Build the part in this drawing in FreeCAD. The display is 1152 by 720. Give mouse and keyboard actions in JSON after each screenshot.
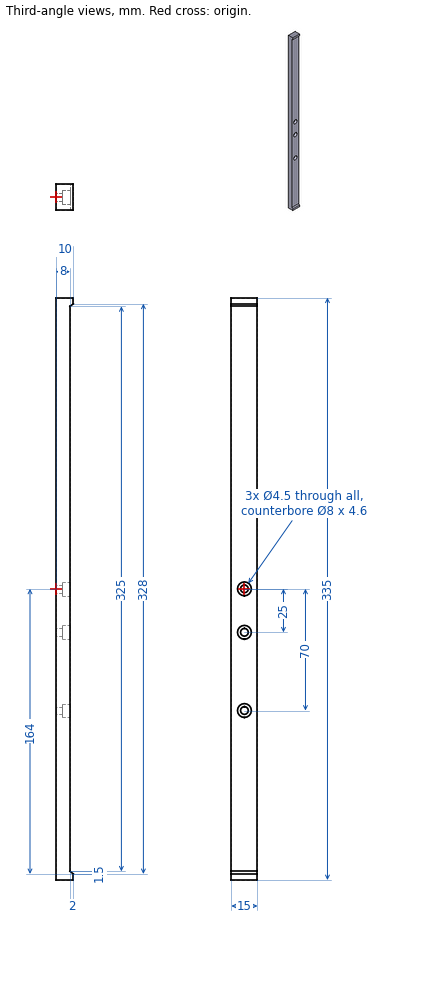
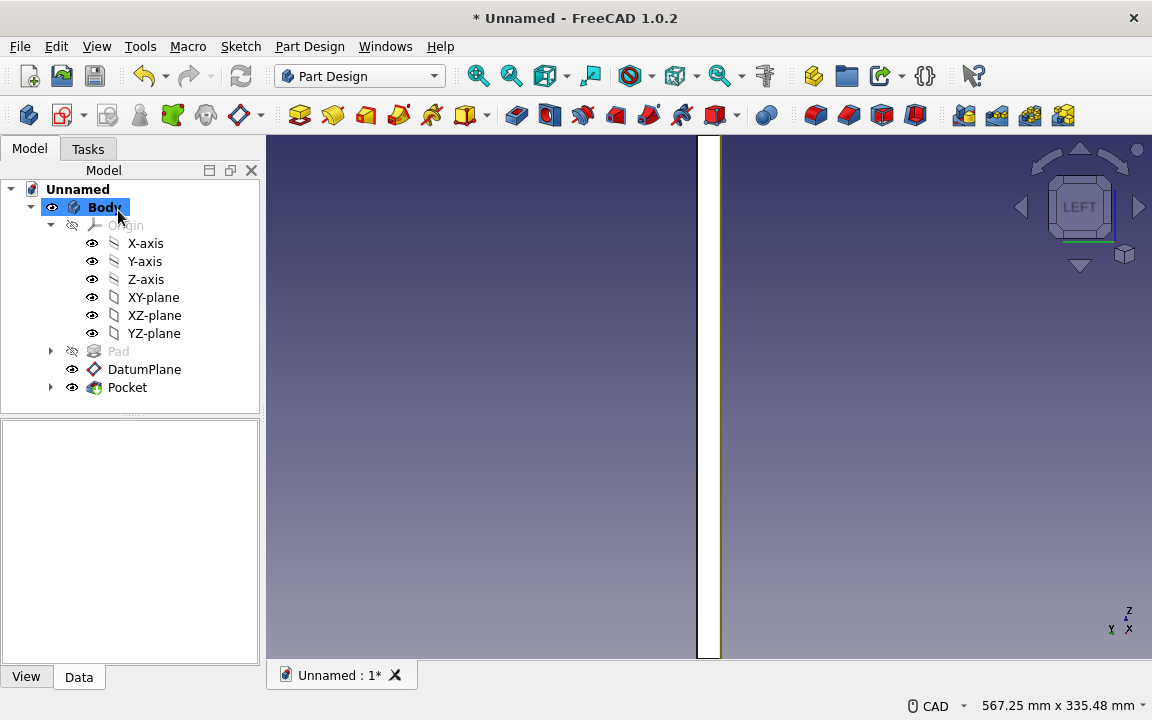
{"action": "left_click", "coordinate": [117, 369]}
{"action": "key", "text": "space"}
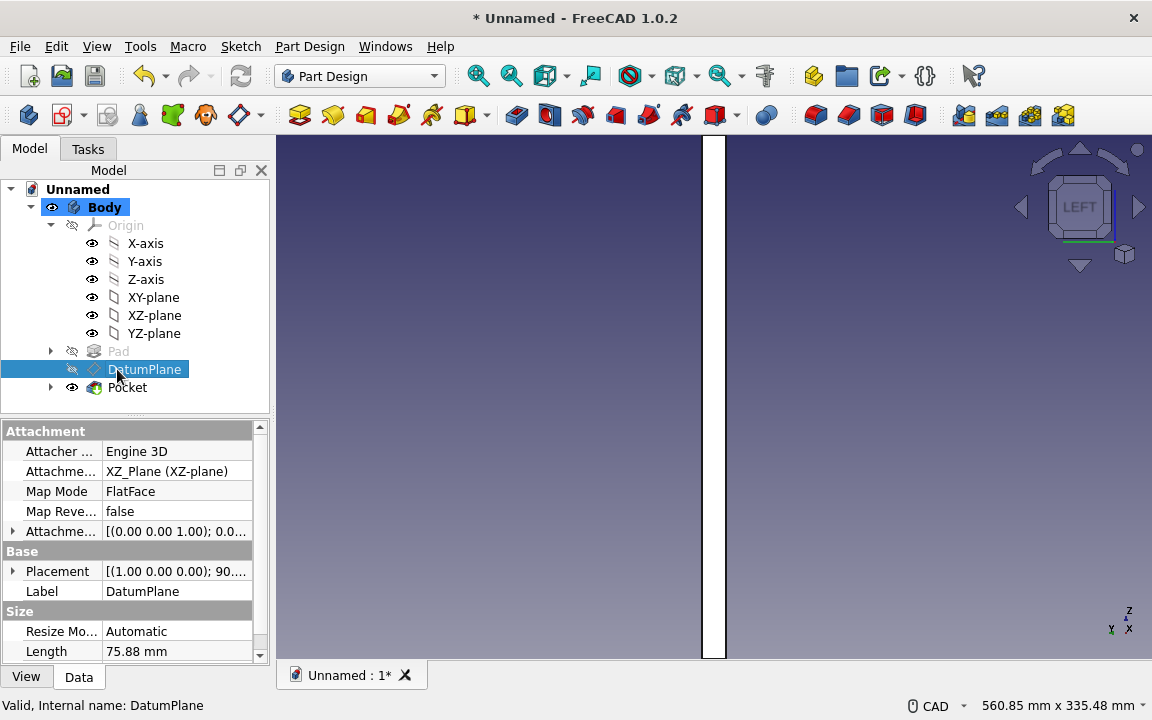
{"action": "left_click", "coordinate": [479, 76]}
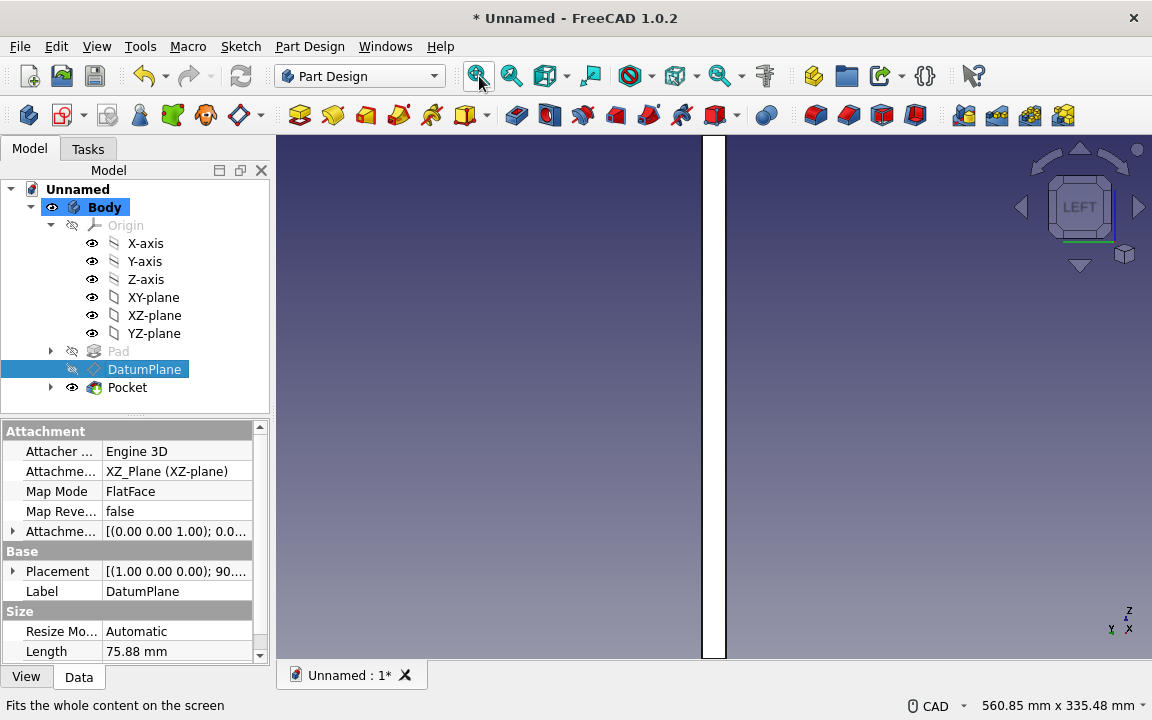
{"action": "key", "text": "0"}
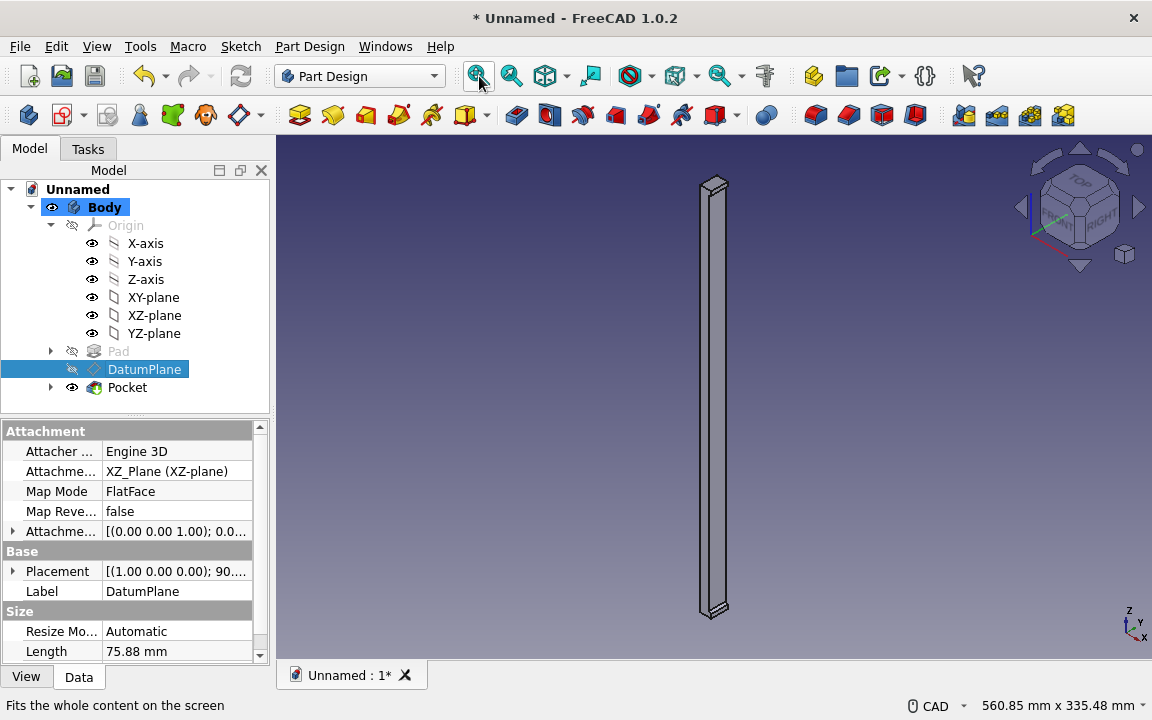
{"action": "key", "text": "3"}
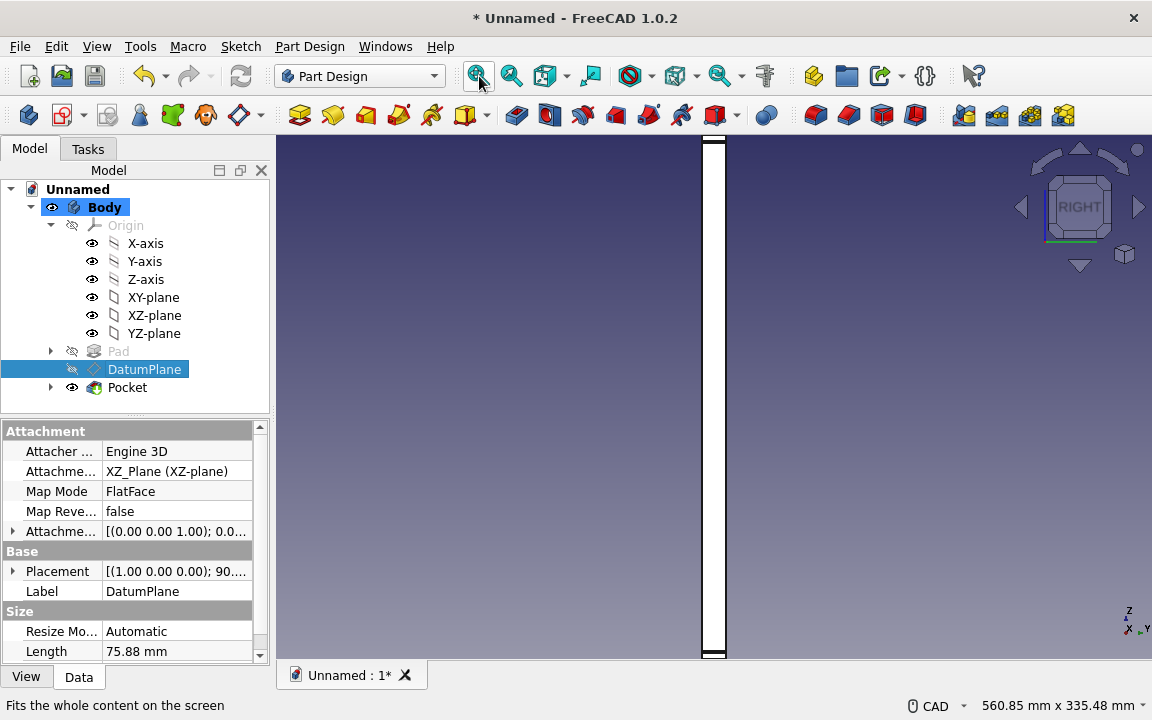
{"action": "left_click", "coordinate": [479, 76]}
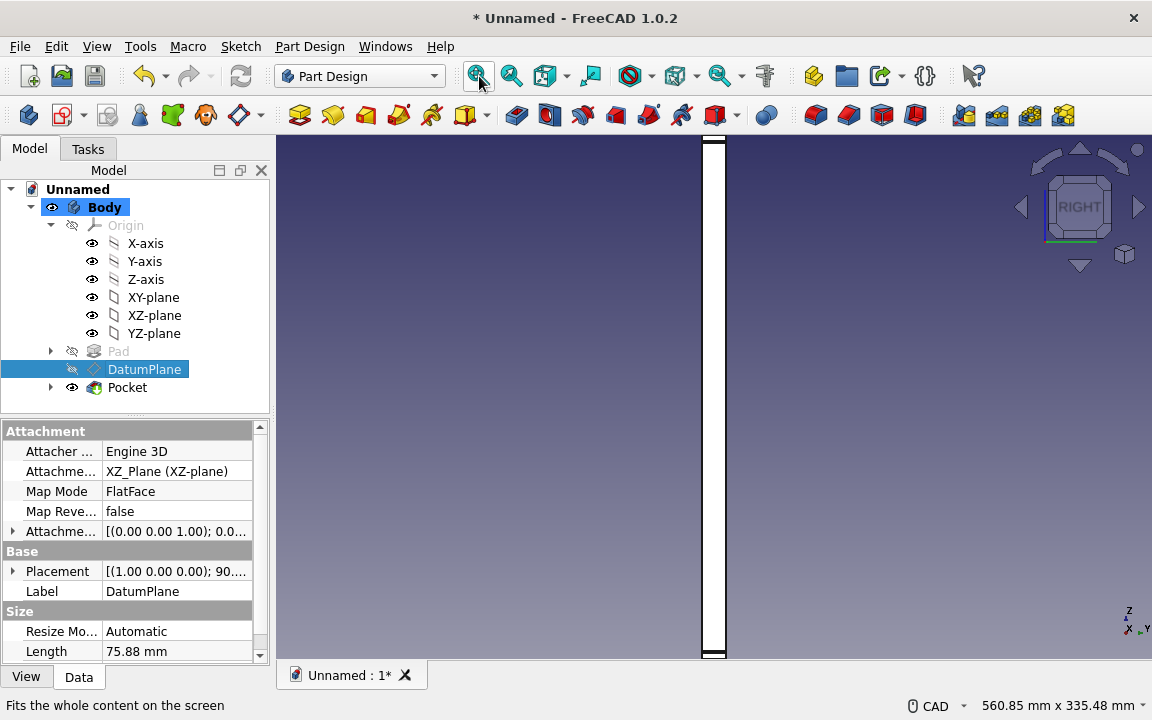
{"action": "left_click", "coordinate": [714, 178]}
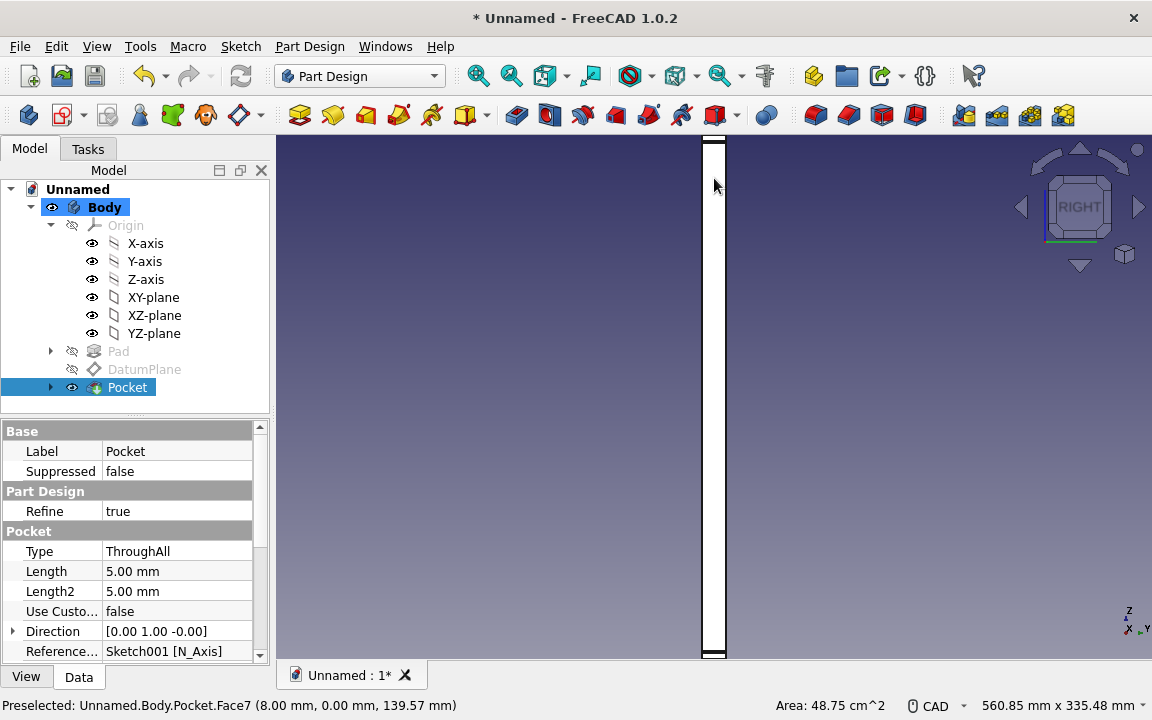
{"action": "left_click", "coordinate": [62, 116]}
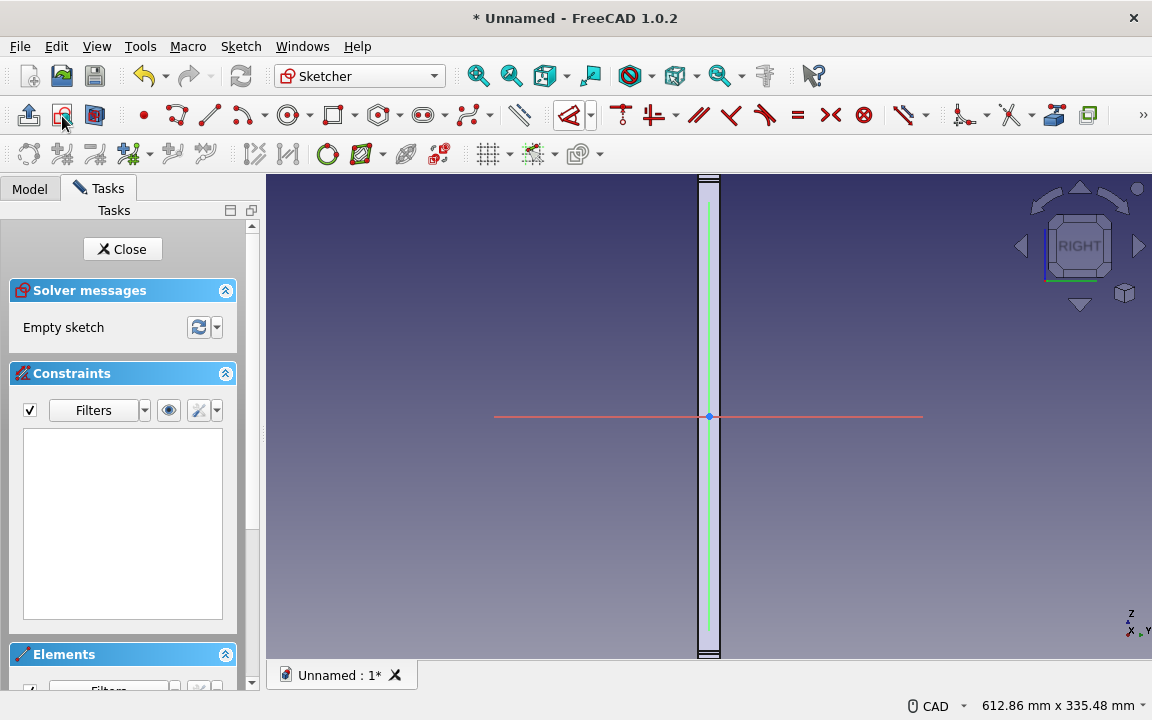
{"action": "left_click", "coordinate": [95, 116]}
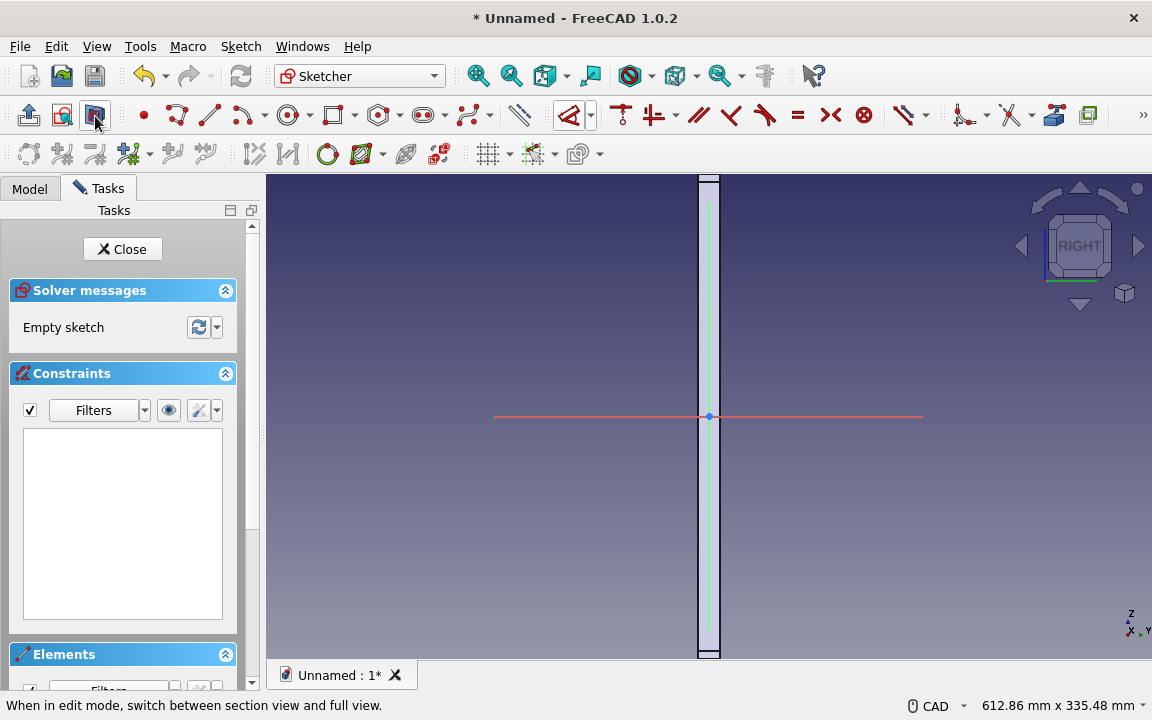
{"action": "scroll", "coordinate": [749, 497], "scroll_direction": "up", "scroll_amount": 5}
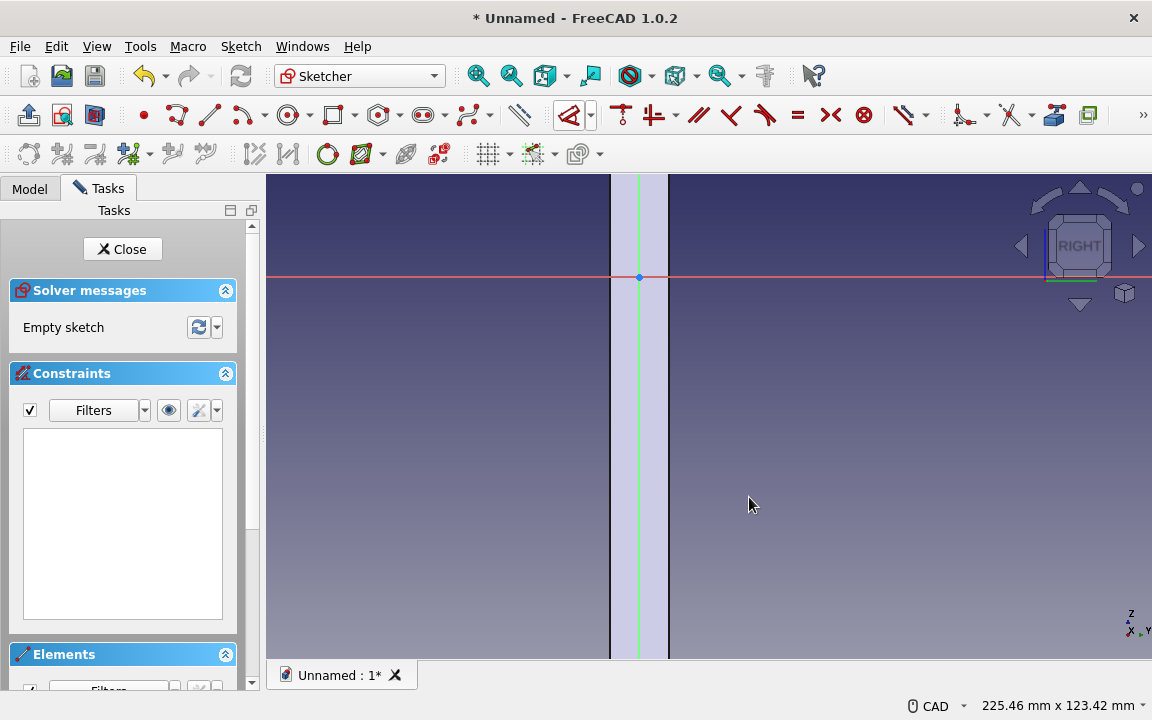
{"action": "left_click", "coordinate": [288, 116]}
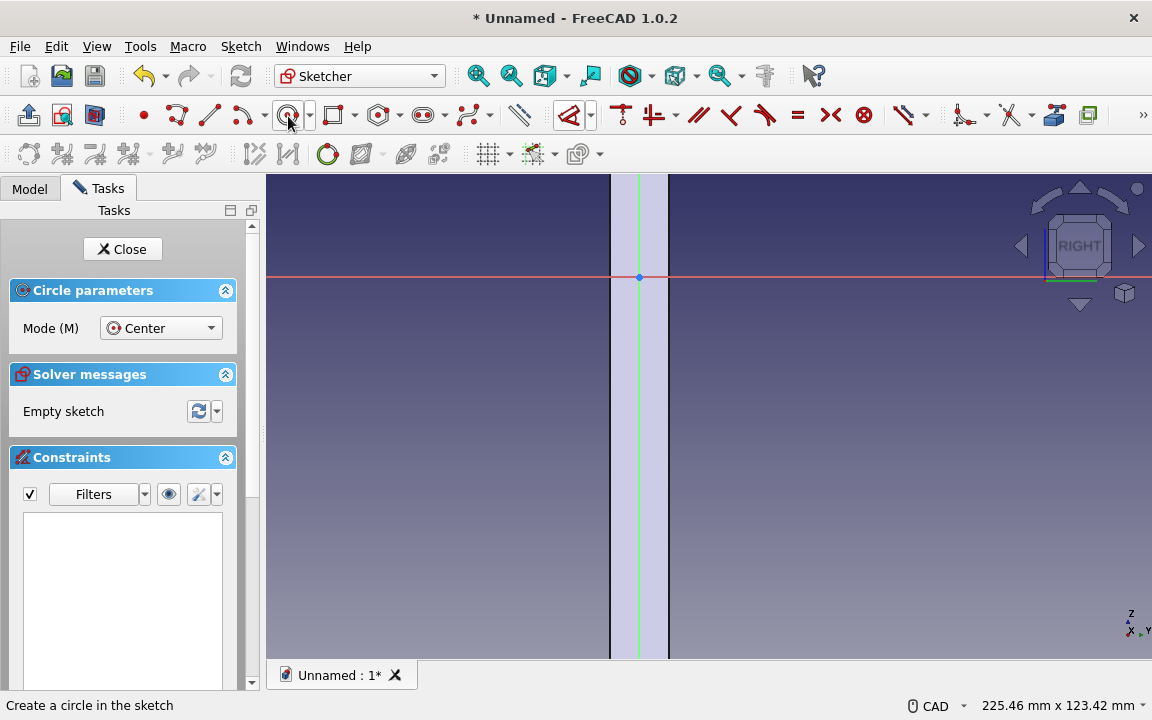
{"action": "scroll", "coordinate": [639, 277], "scroll_direction": "up", "scroll_amount": 5}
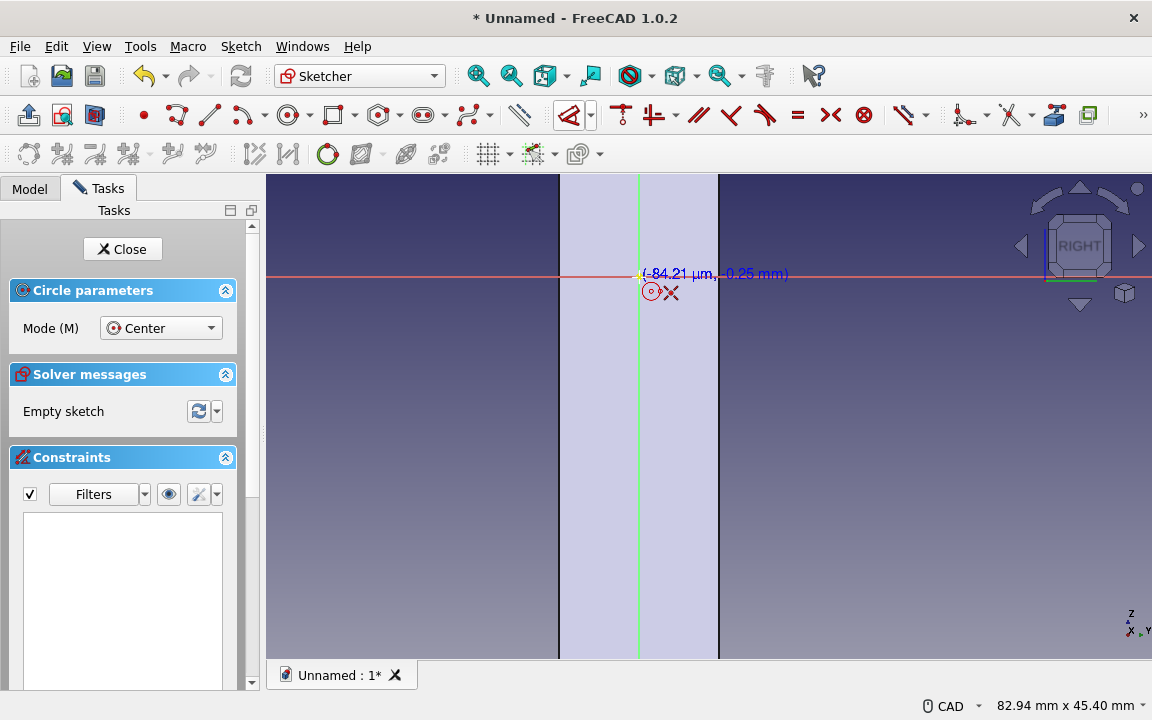
{"action": "left_click", "coordinate": [639, 277]}
{"action": "left_click", "coordinate": [656, 260]}